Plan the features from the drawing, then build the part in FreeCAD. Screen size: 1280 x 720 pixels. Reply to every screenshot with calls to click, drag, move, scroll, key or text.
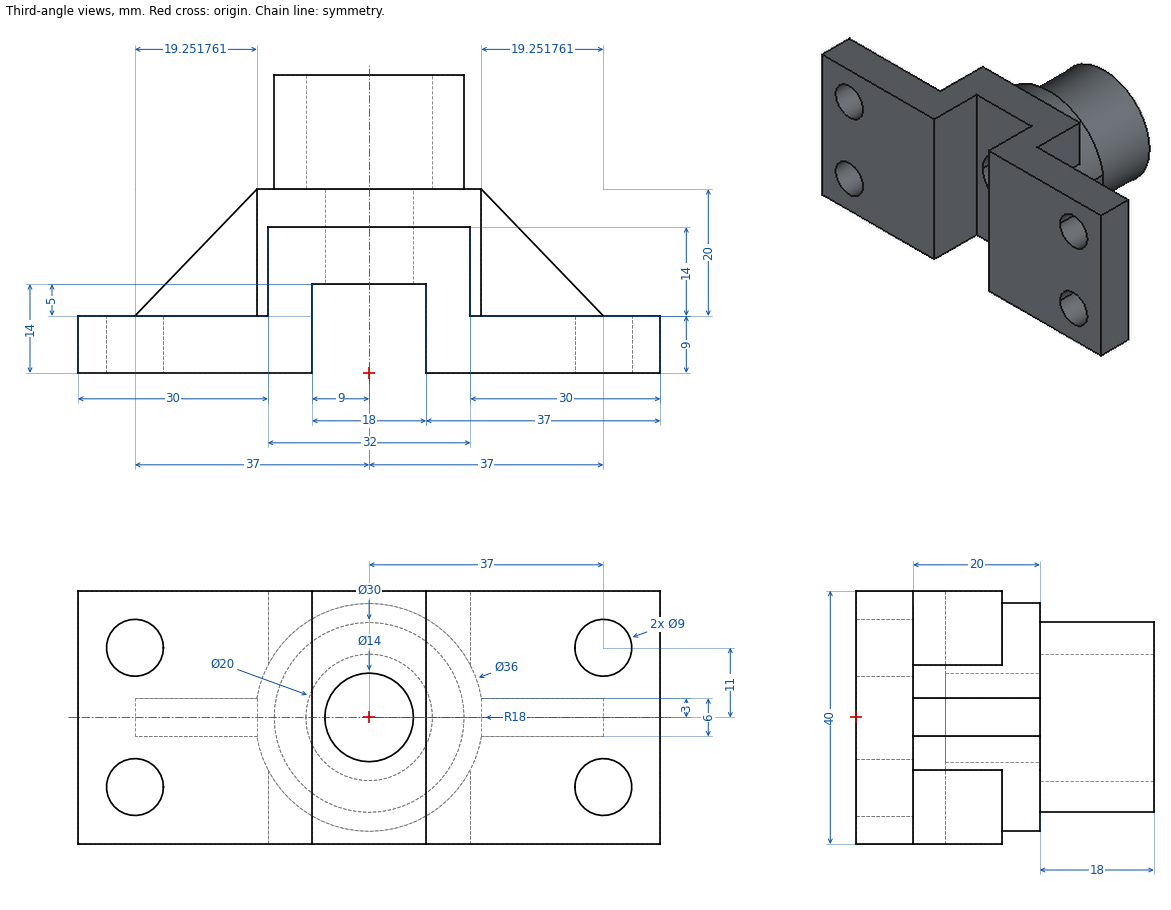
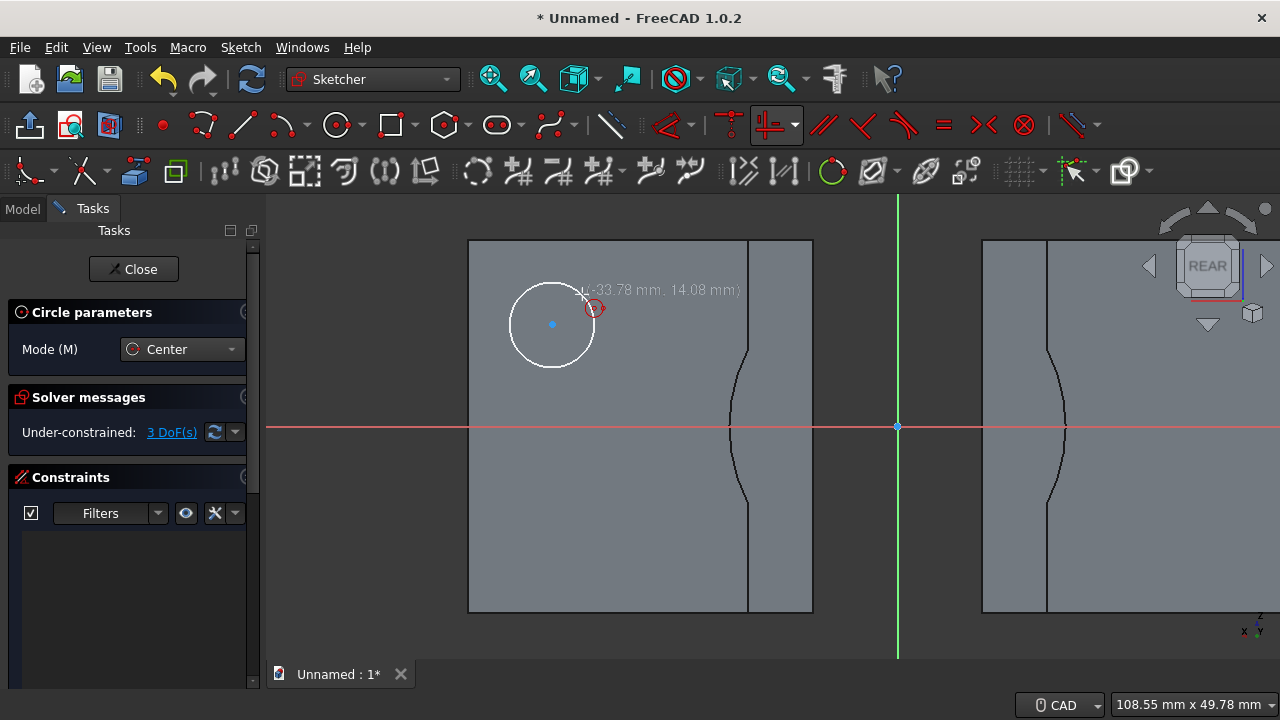
click(552, 529)
click(582, 500)
key(Escape)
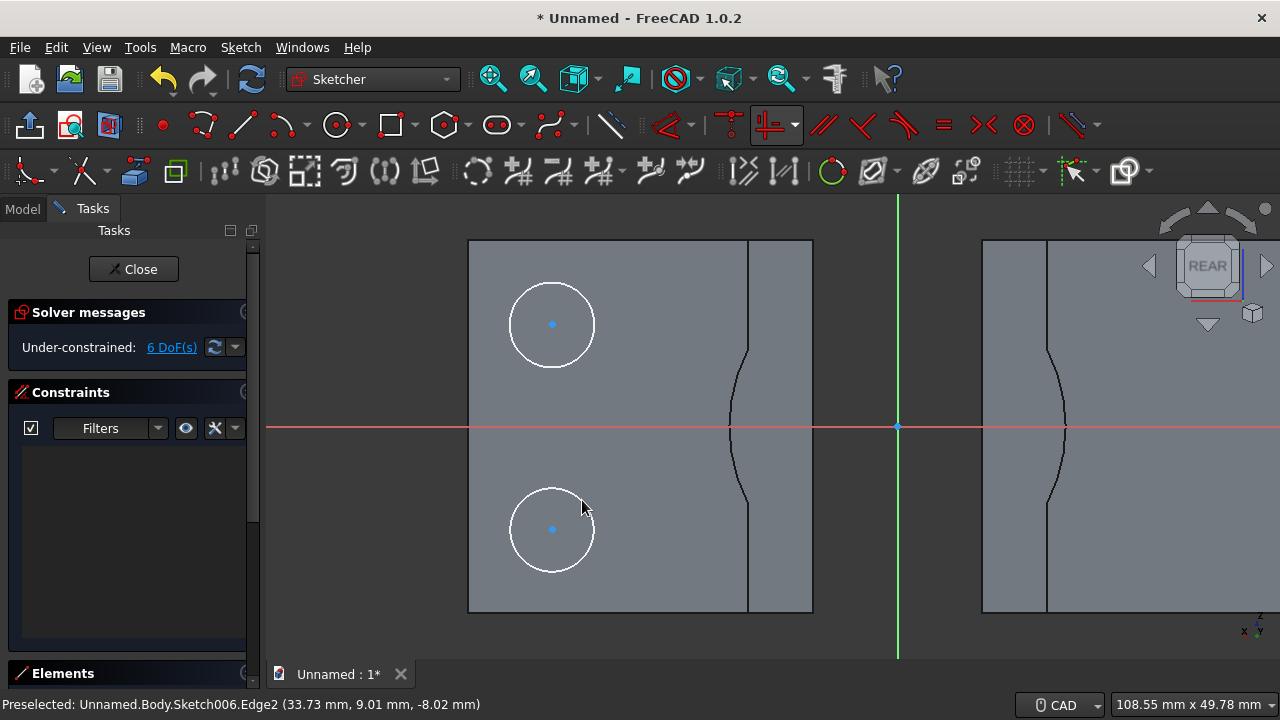
click(582, 295)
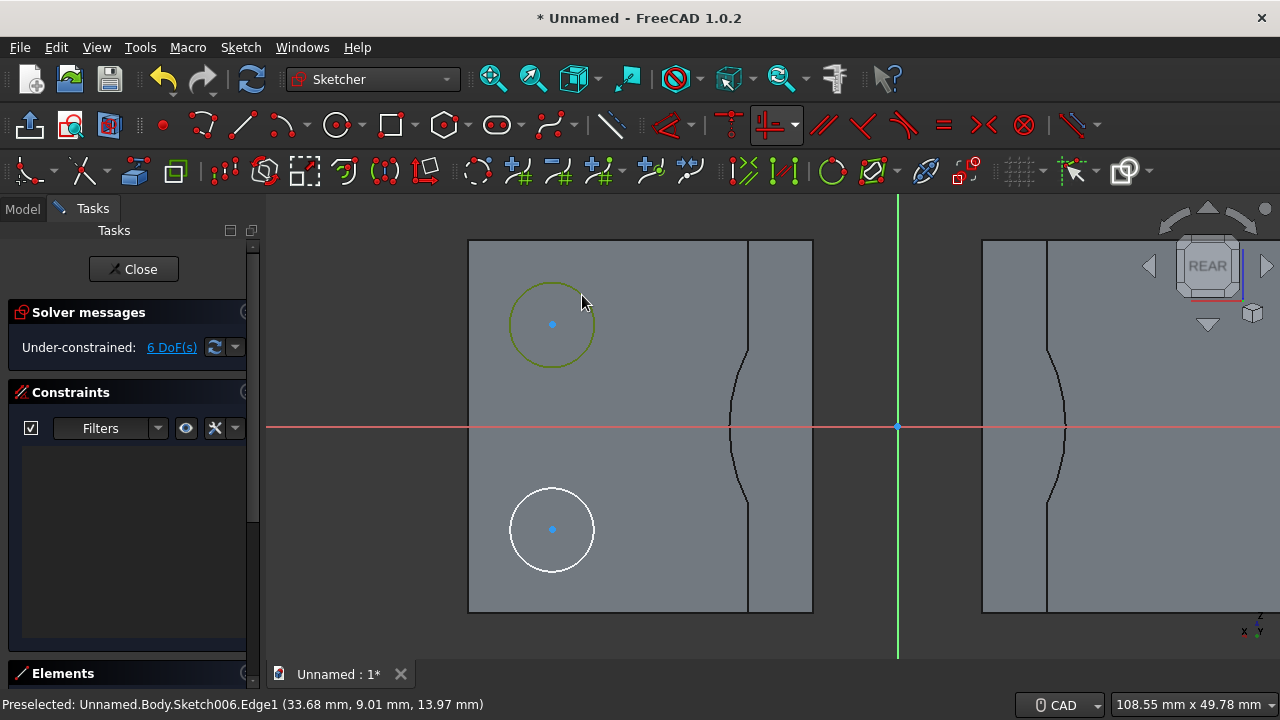
click(581, 500)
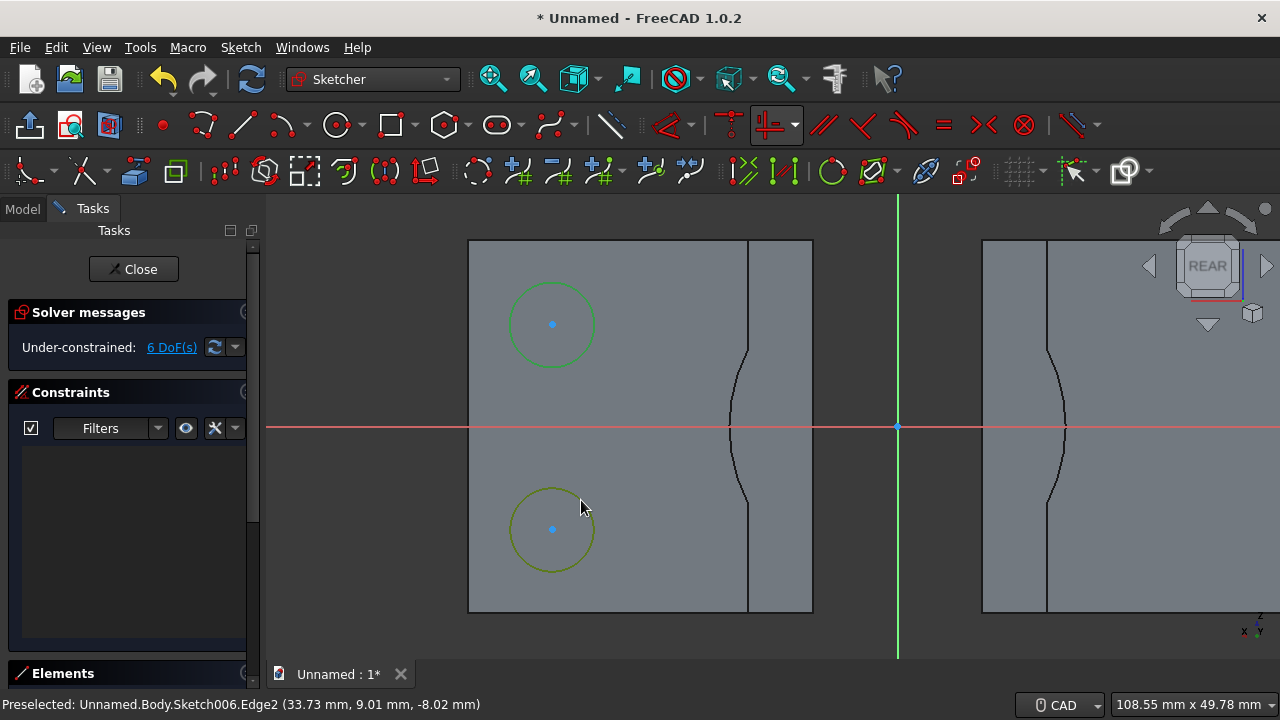
key(e)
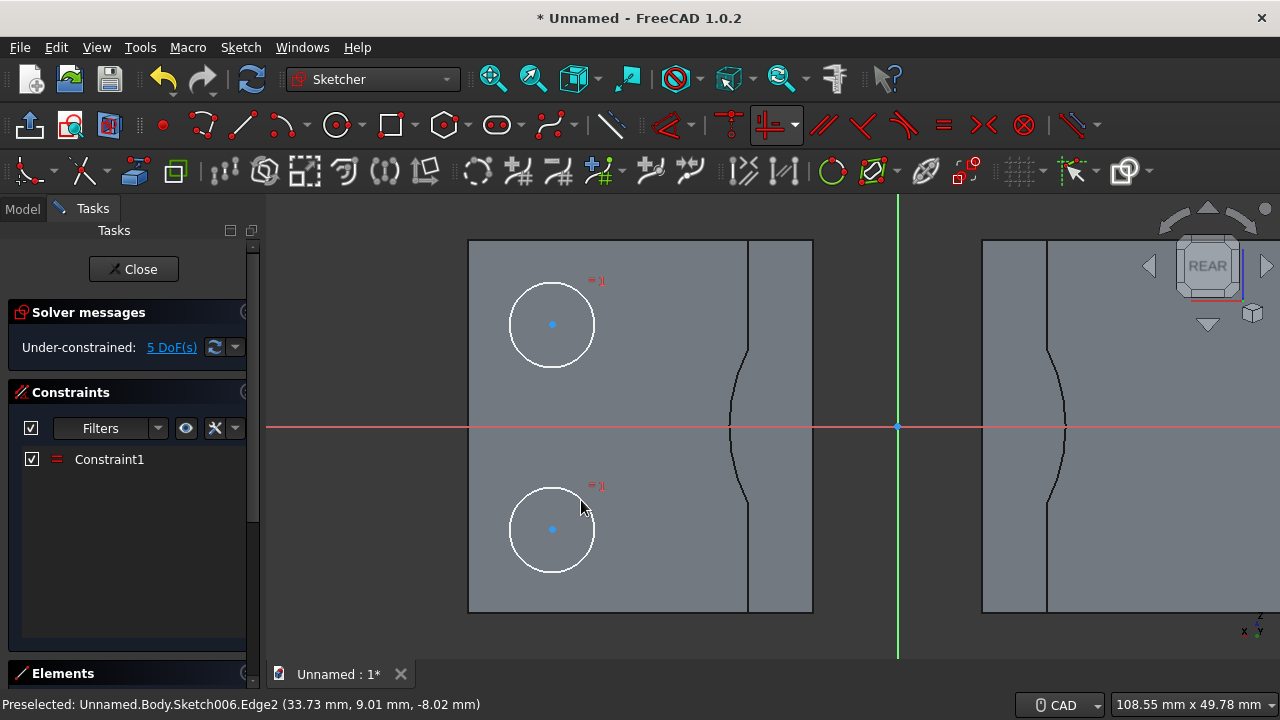
click(552, 325)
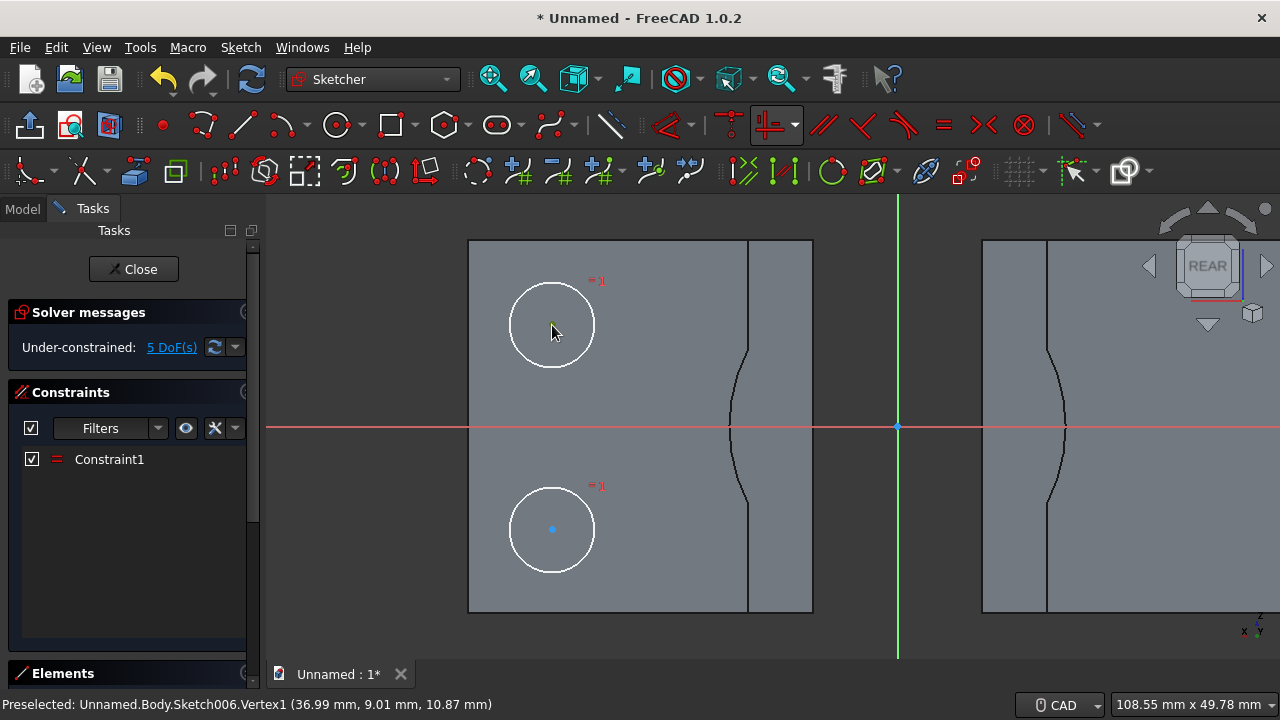
click(552, 530)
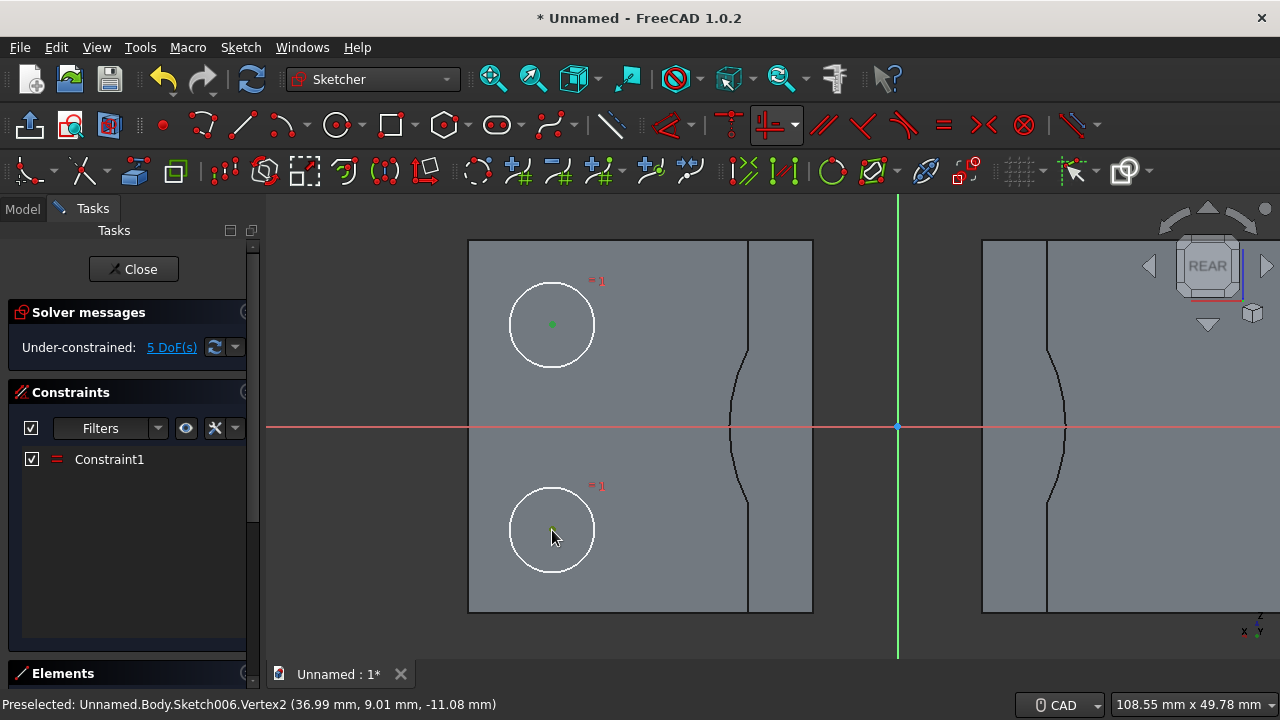
click(353, 426)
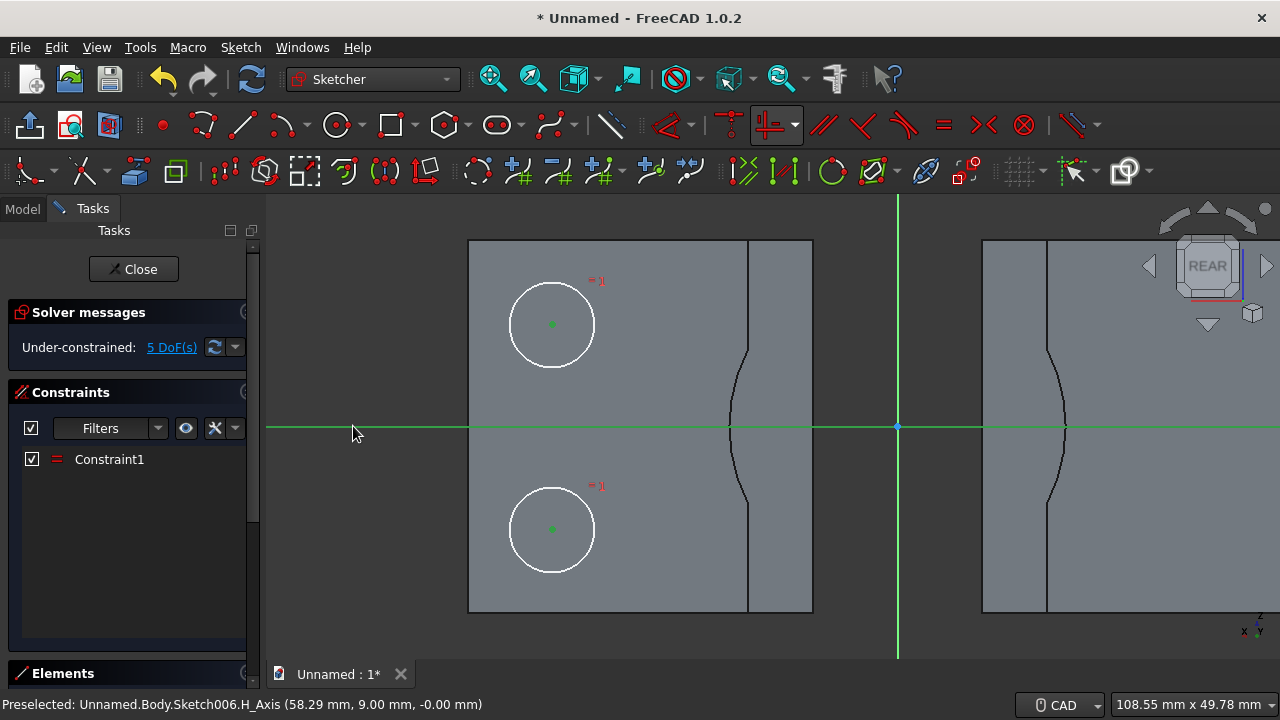
key(s)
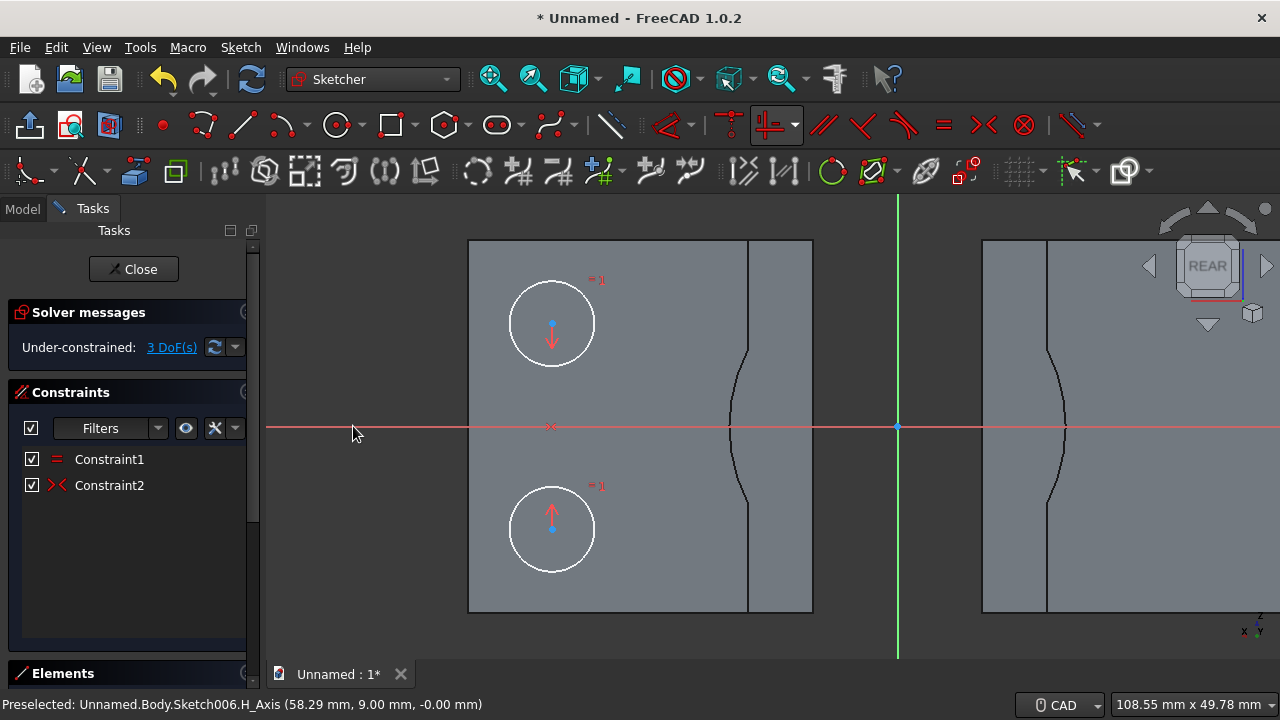
click(666, 126)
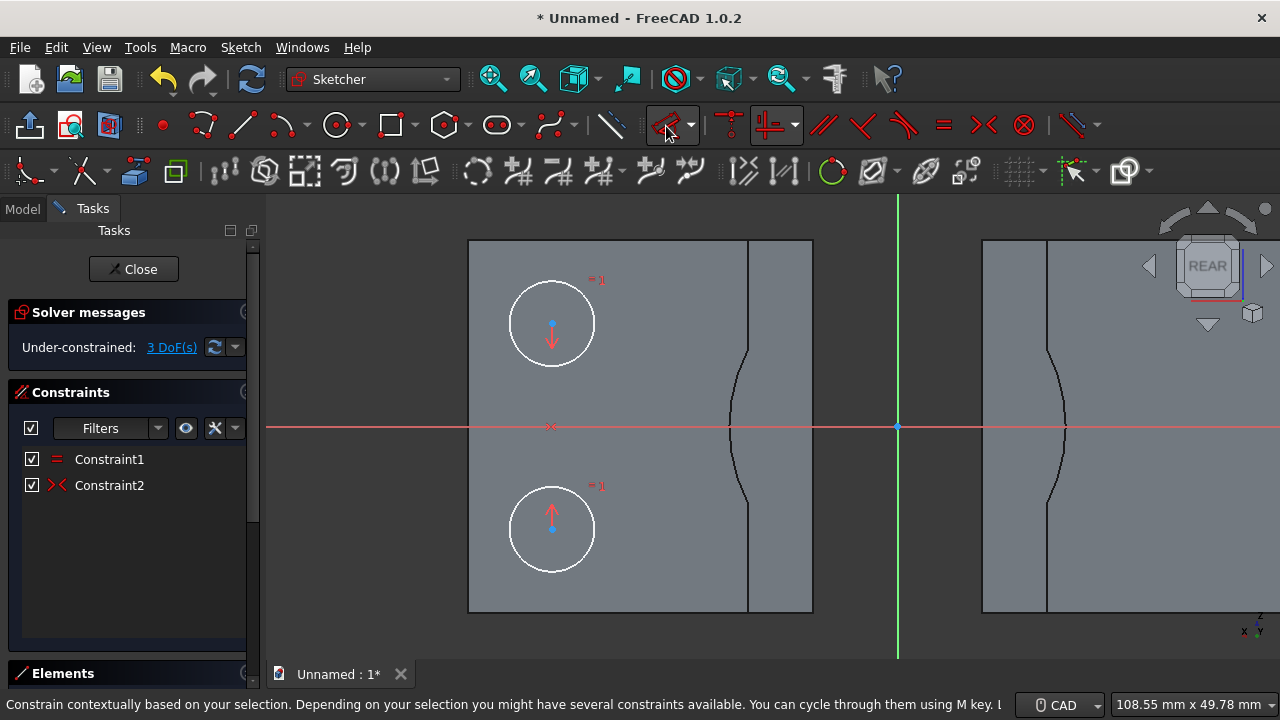
click(582, 294)
click(605, 272)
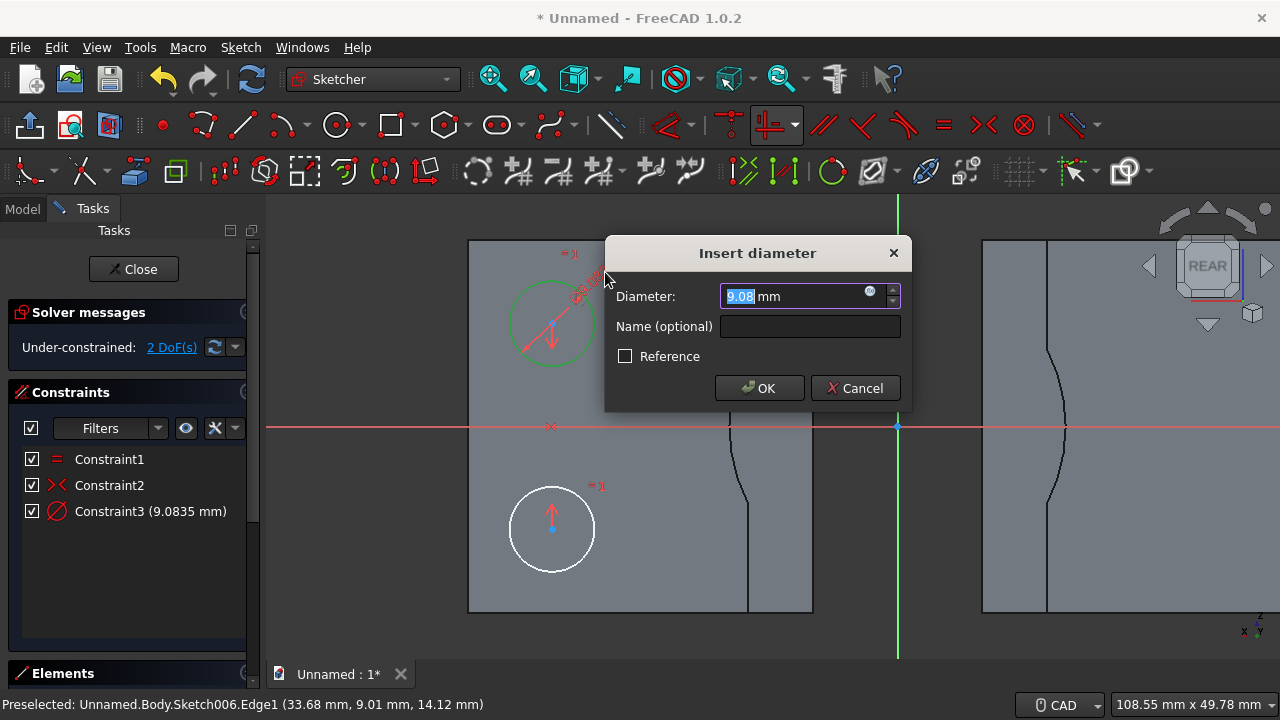
text(9)
key(Return)